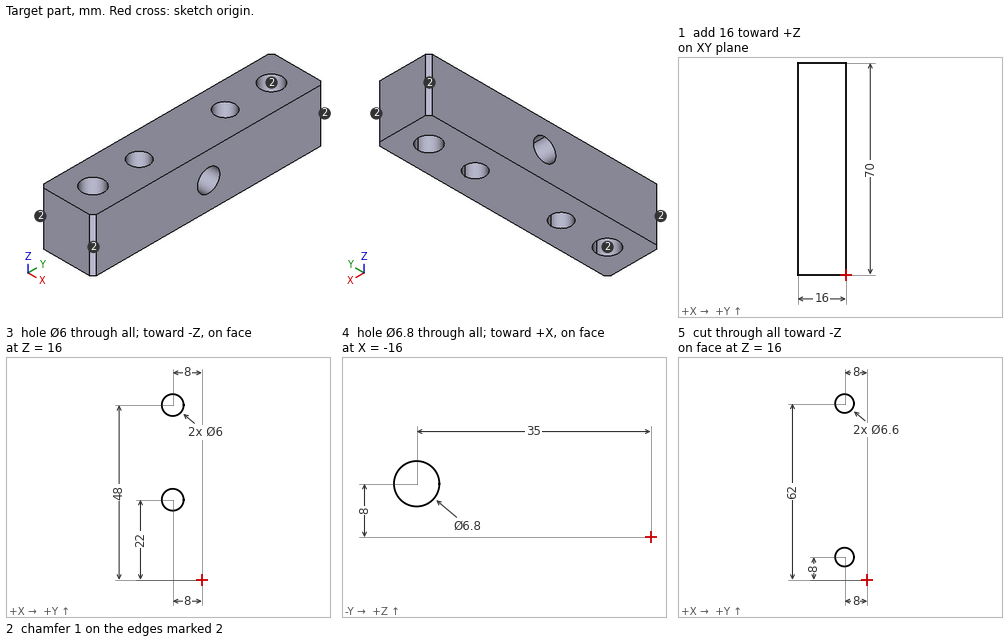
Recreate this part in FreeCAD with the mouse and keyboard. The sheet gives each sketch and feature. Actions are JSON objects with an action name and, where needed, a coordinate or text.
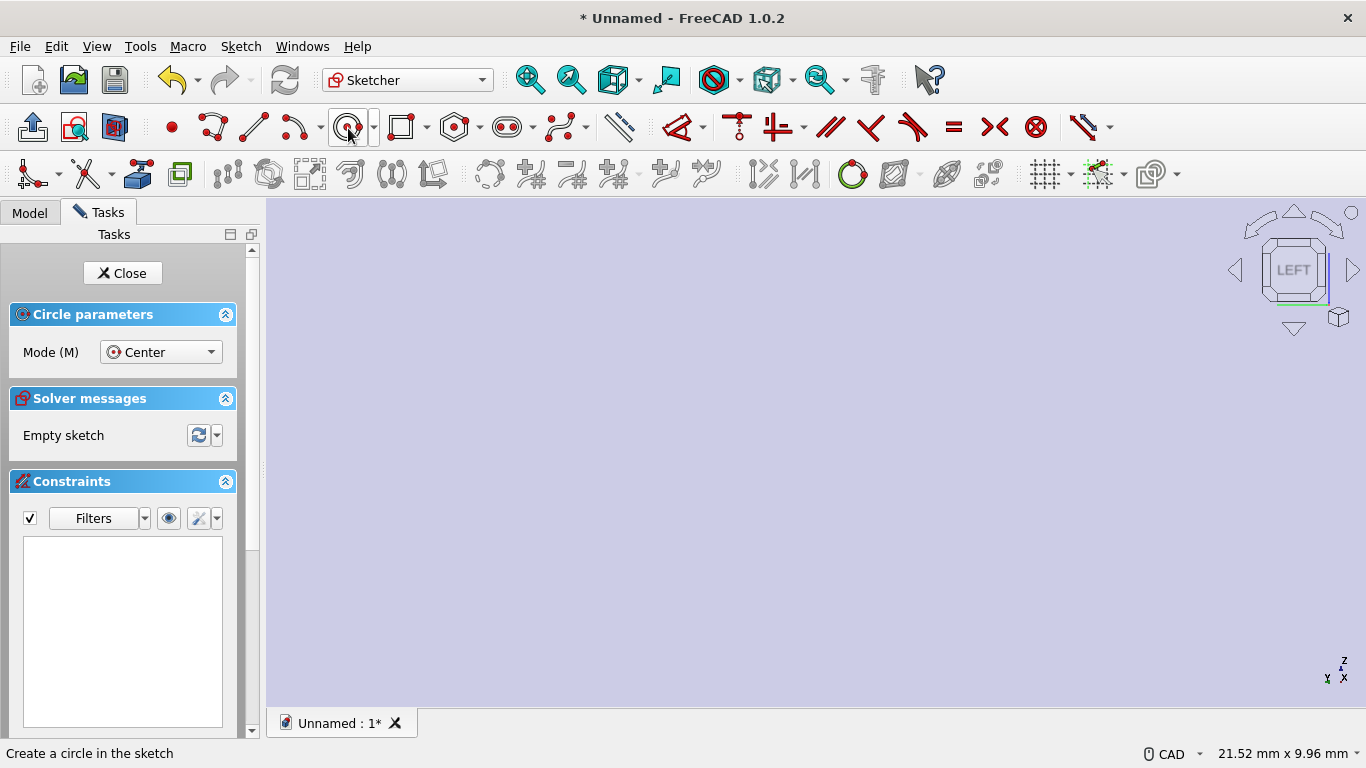
{"action": "left_click", "coordinate": [742, 452]}
{"action": "mouse_move", "coordinate": [865, 330]}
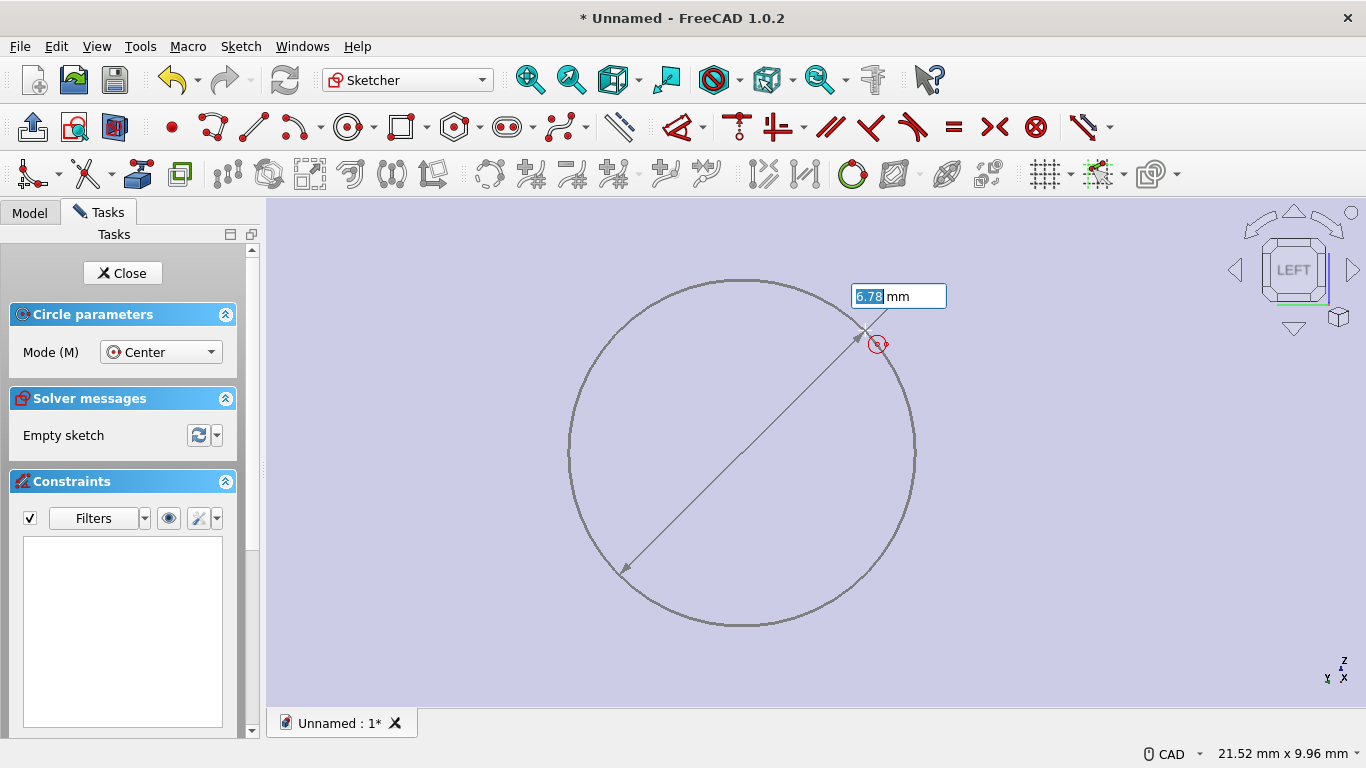
{"action": "type", "text": "6.8"}
{"action": "key", "text": "Return"}
{"action": "key", "text": "Escape"}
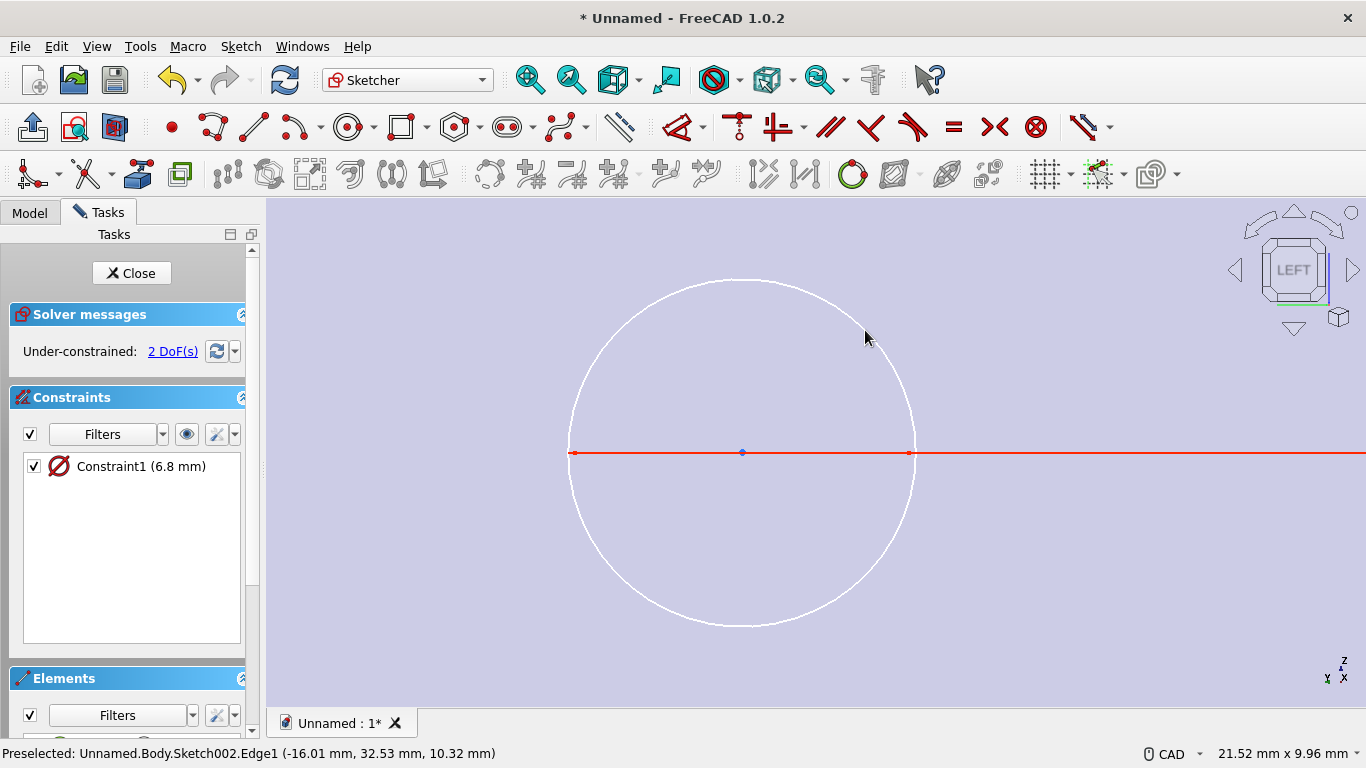
{"action": "key", "text": "d"}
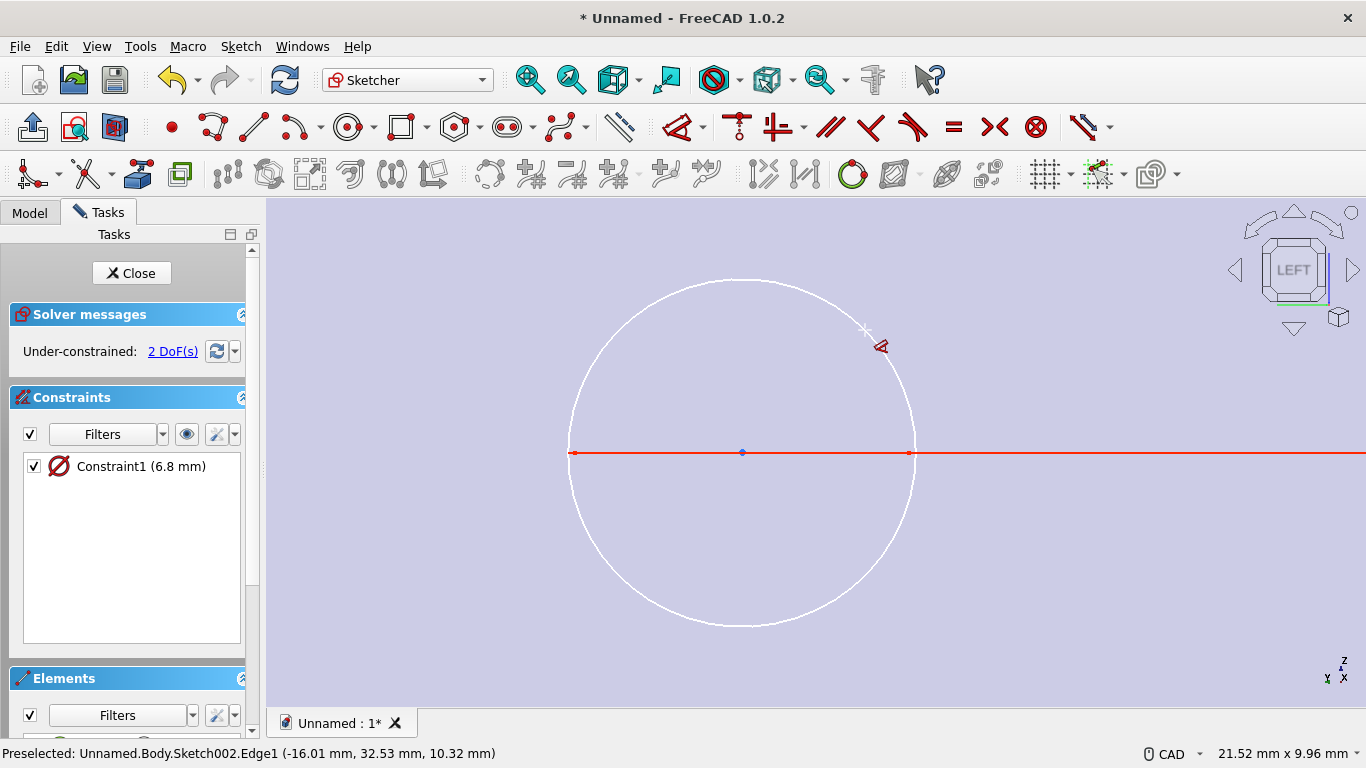
{"action": "left_click", "coordinate": [742, 453]}
{"action": "left_click", "coordinate": [708, 566]}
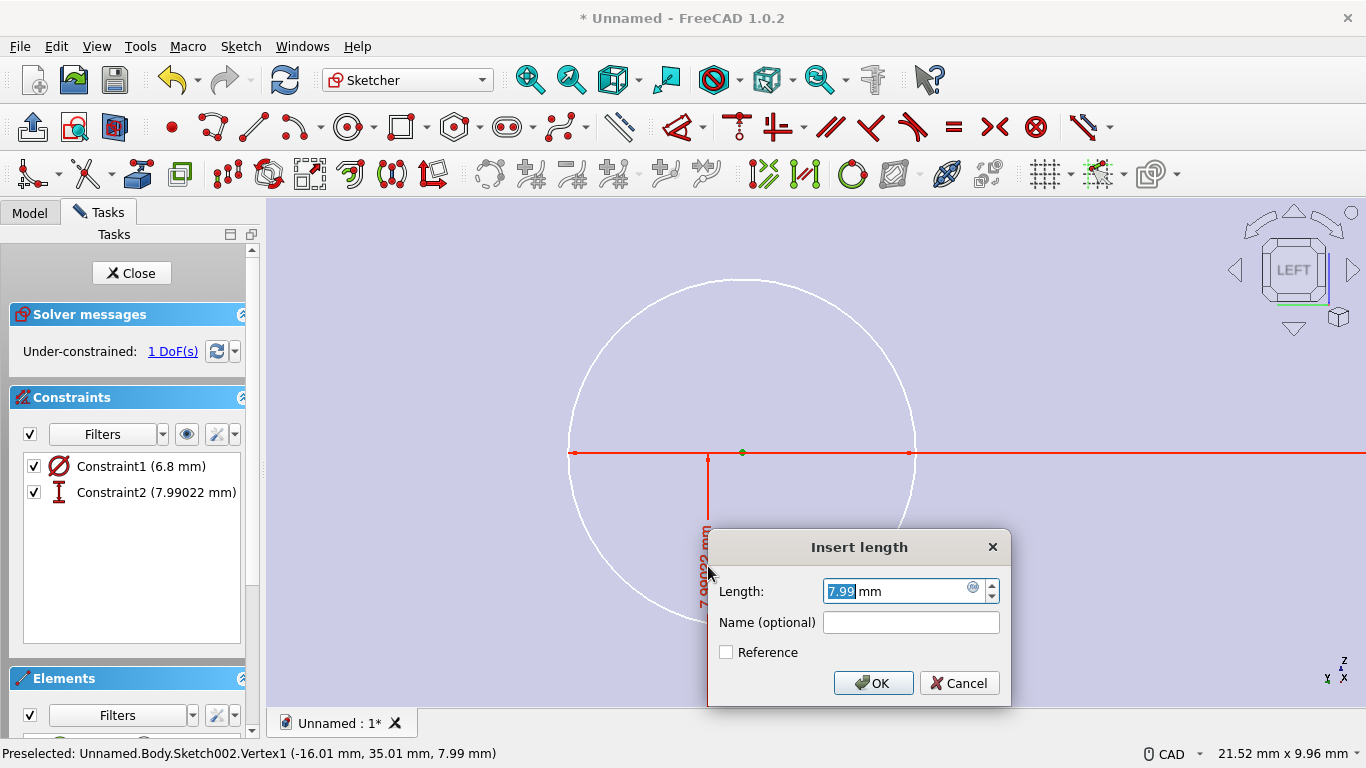
{"action": "type", "text": "8"}
{"action": "key", "text": "Return"}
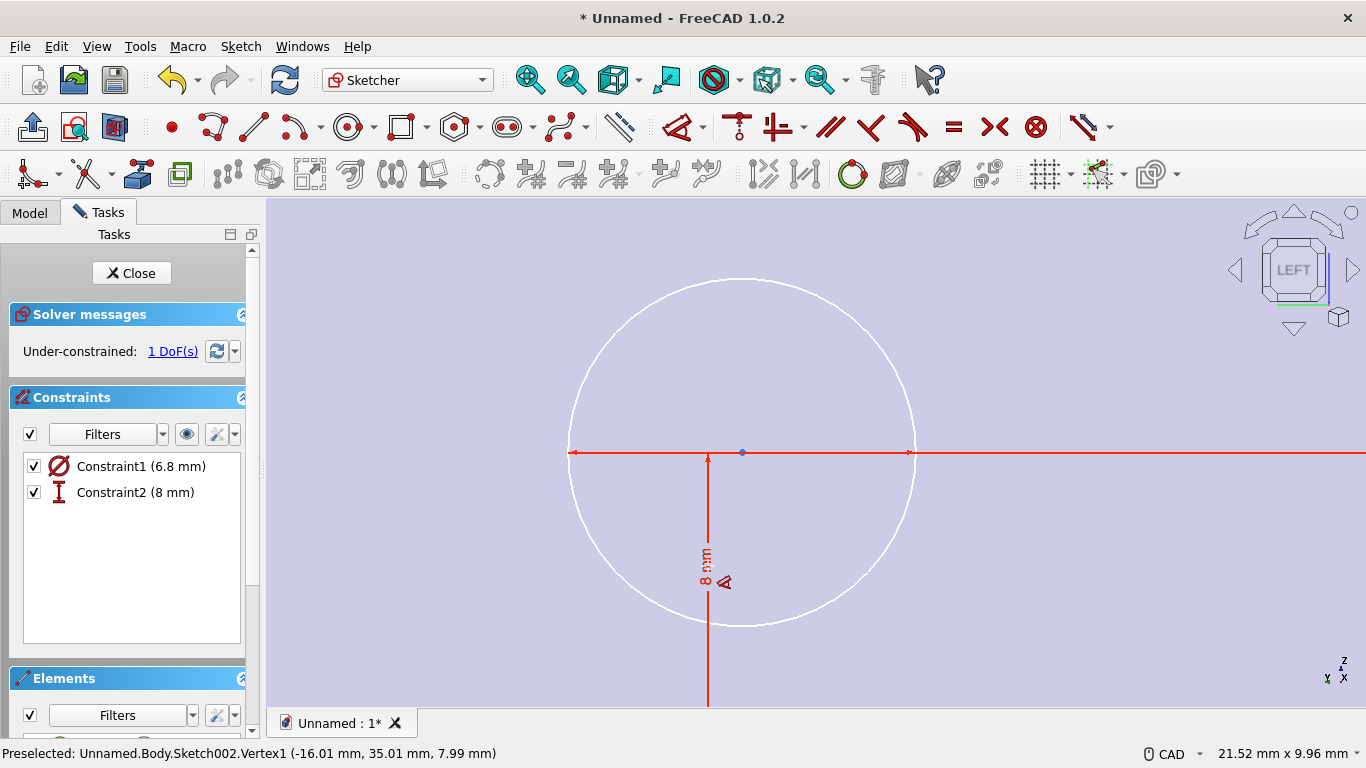
{"action": "left_click", "coordinate": [742, 452]}
{"action": "left_click", "coordinate": [971, 418]}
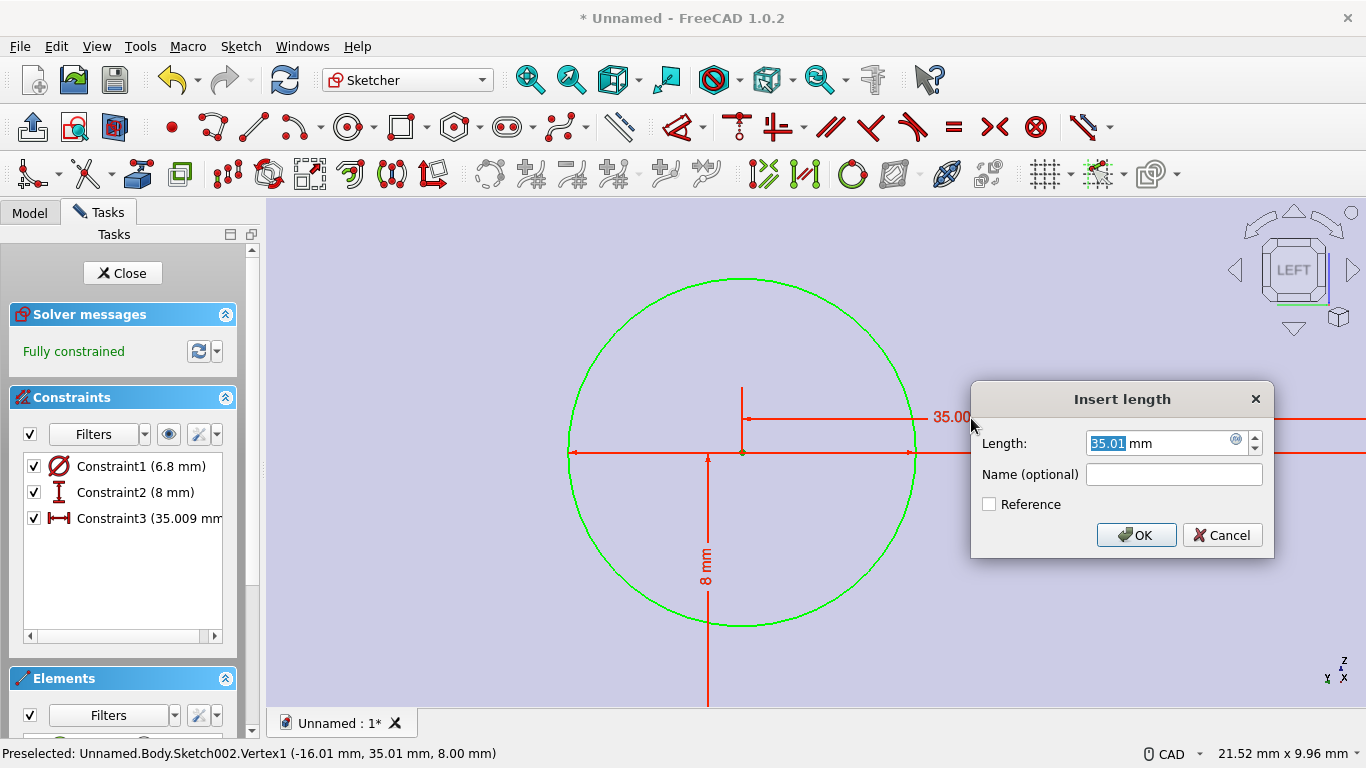
{"action": "type", "text": "35"}
{"action": "key", "text": "Return"}
{"action": "key", "text": "Escape"}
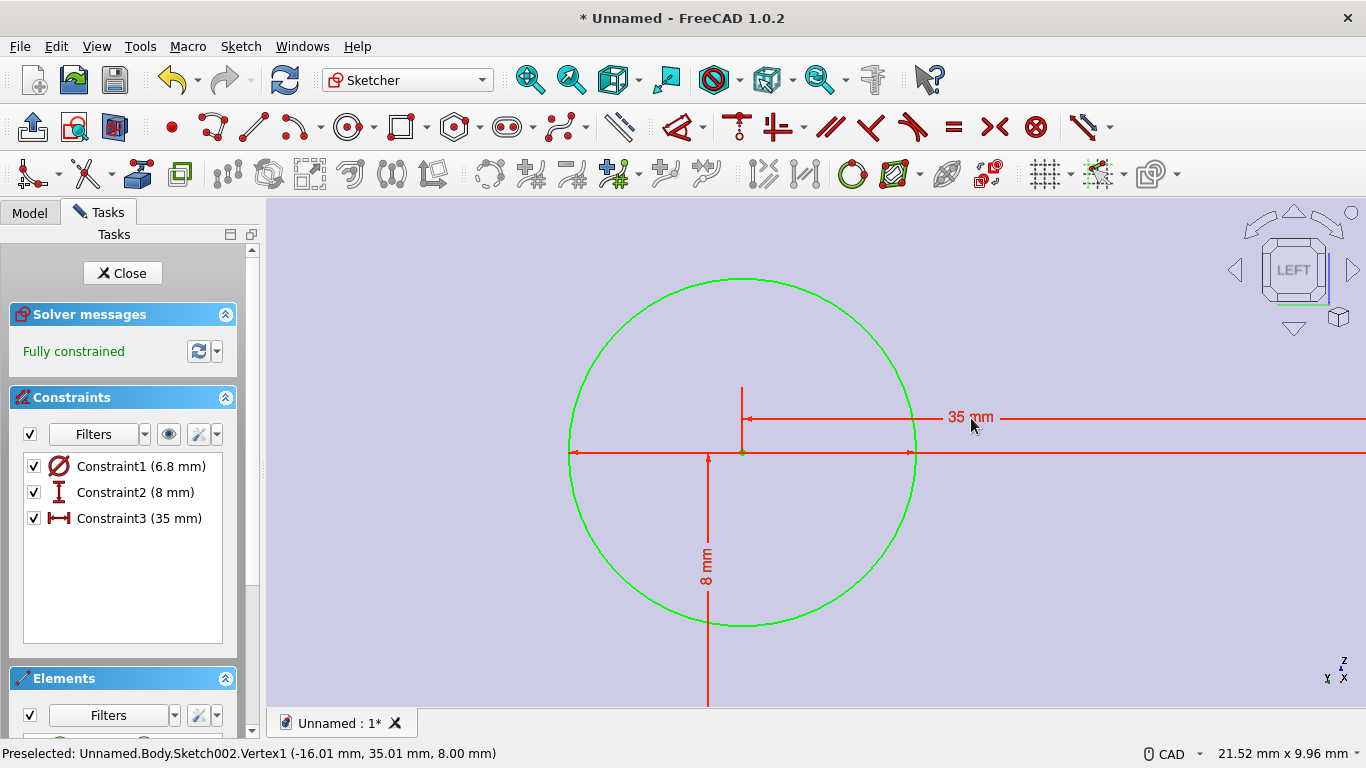
{"action": "left_click", "coordinate": [123, 273]}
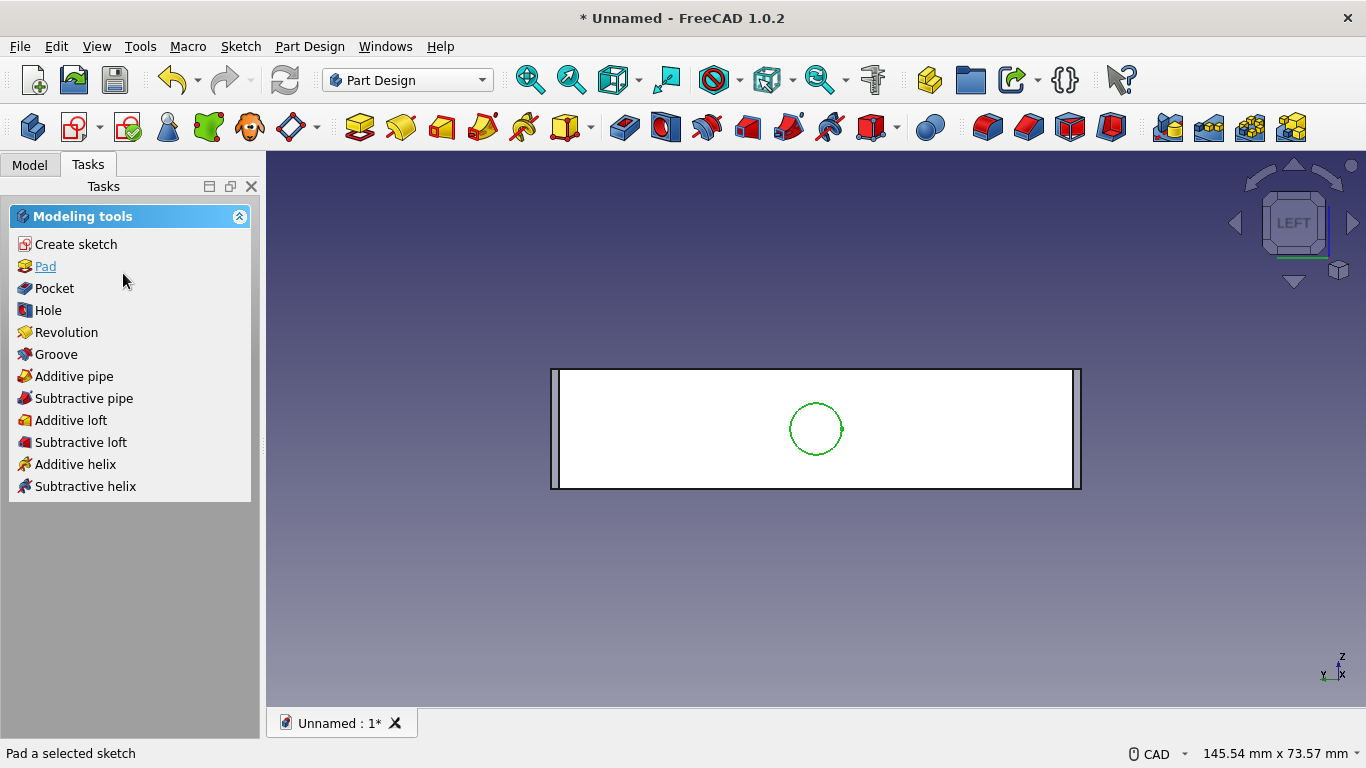
{"action": "left_click", "coordinate": [666, 128]}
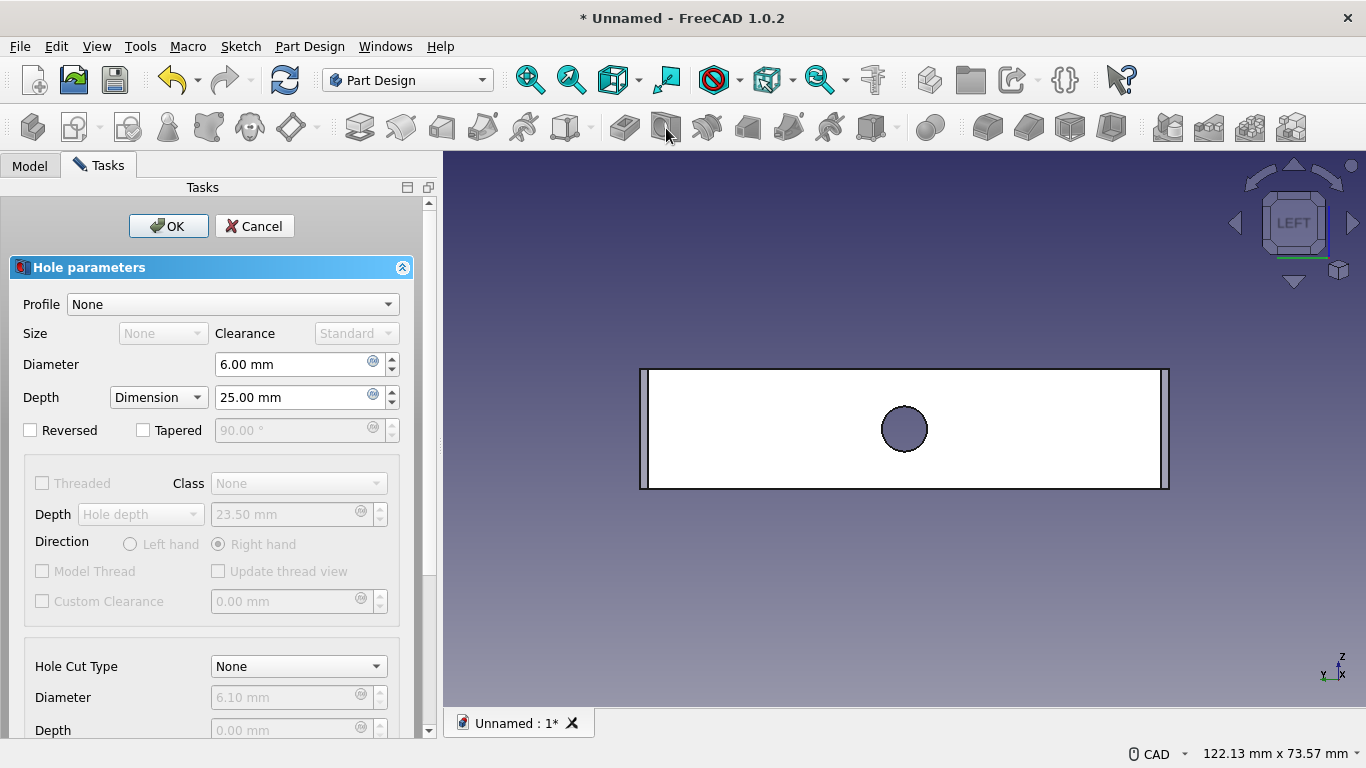
{"action": "triple_click", "coordinate": [300, 364]}